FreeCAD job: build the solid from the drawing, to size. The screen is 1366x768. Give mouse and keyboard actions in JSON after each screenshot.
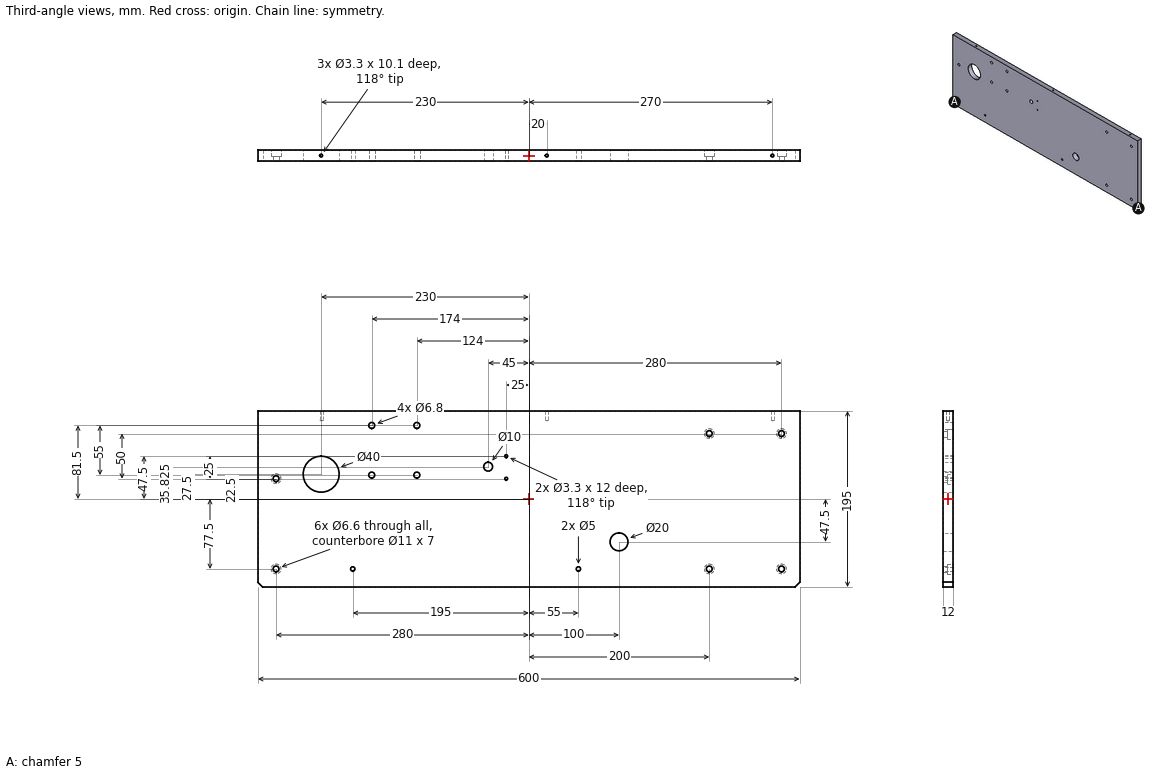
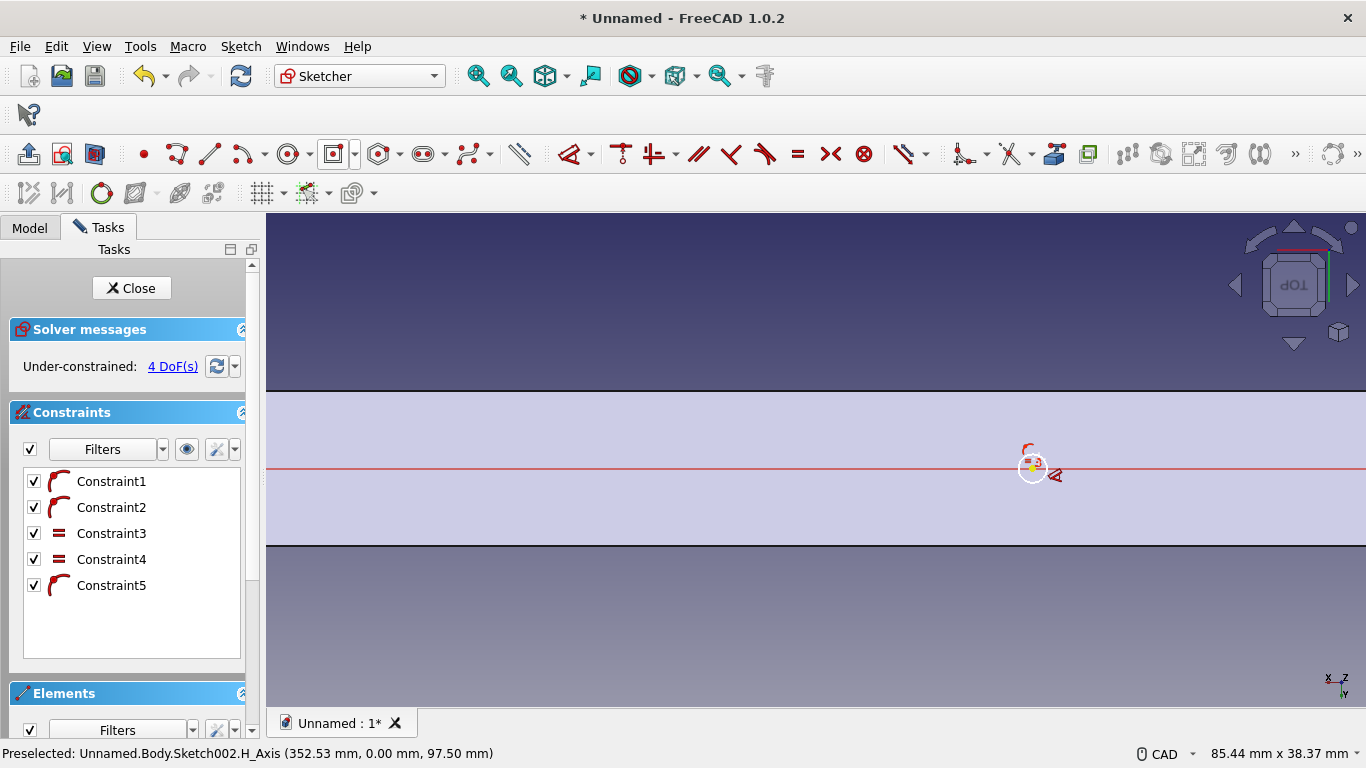
{"action": "left_click", "coordinate": [1033, 454]}
{"action": "left_click", "coordinate": [1034, 422]}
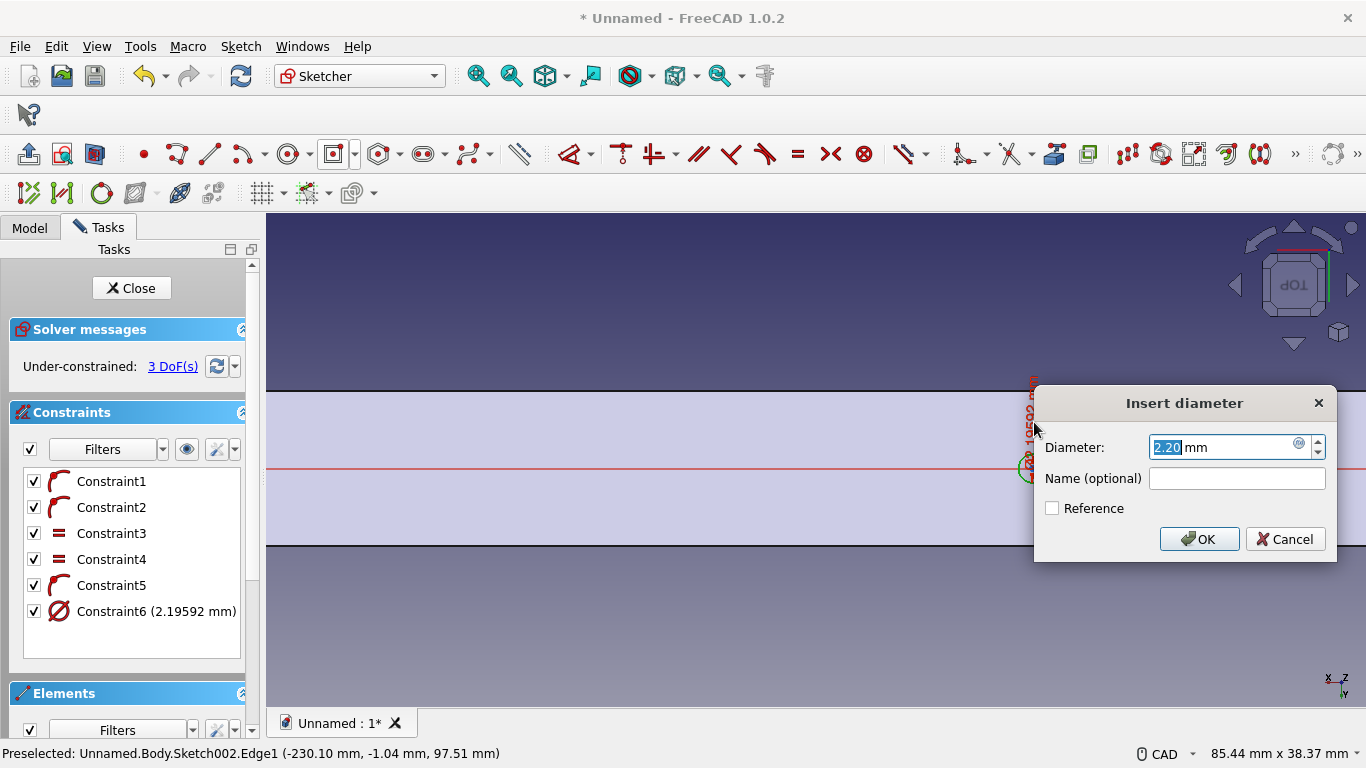
{"action": "type", "text": "3.3"}
{"action": "key", "text": "Return"}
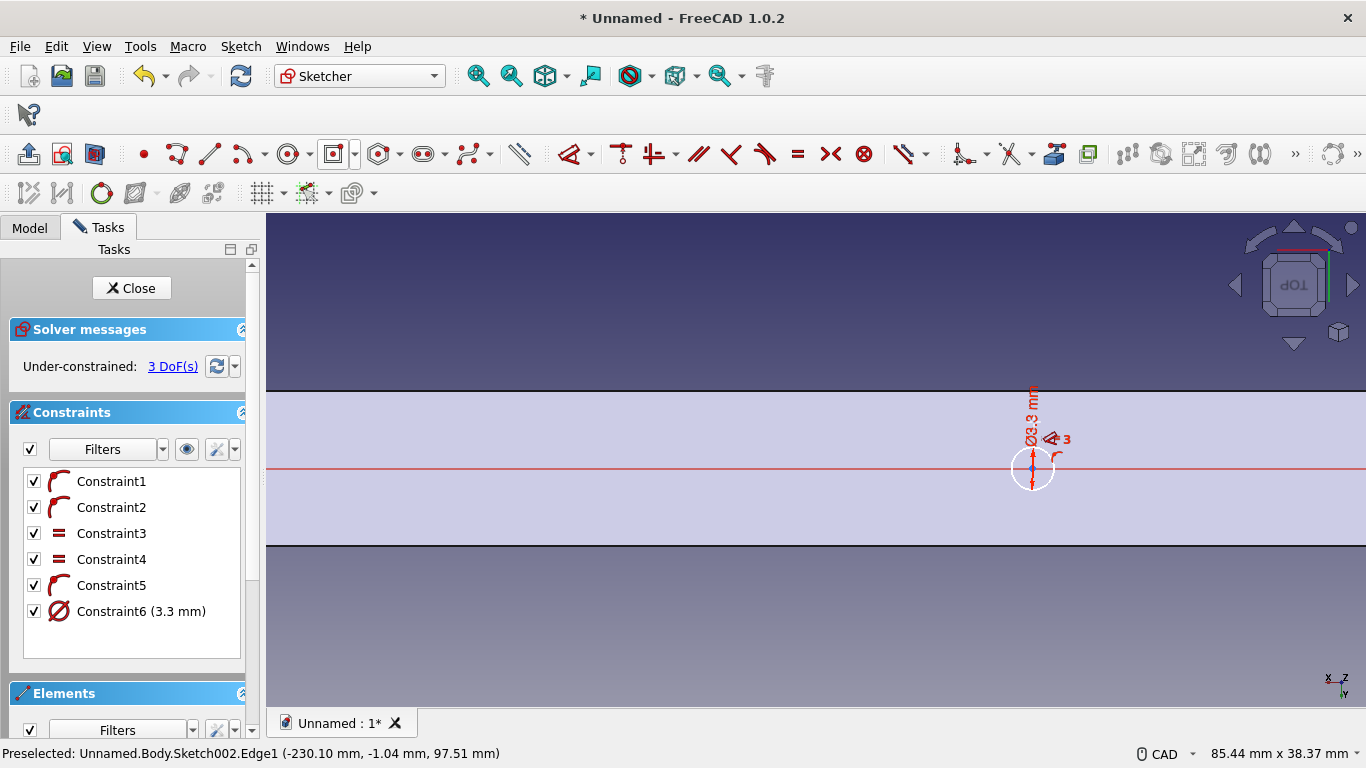
{"action": "scroll", "coordinate": [1040, 459], "scroll_direction": "down", "scroll_amount": 12}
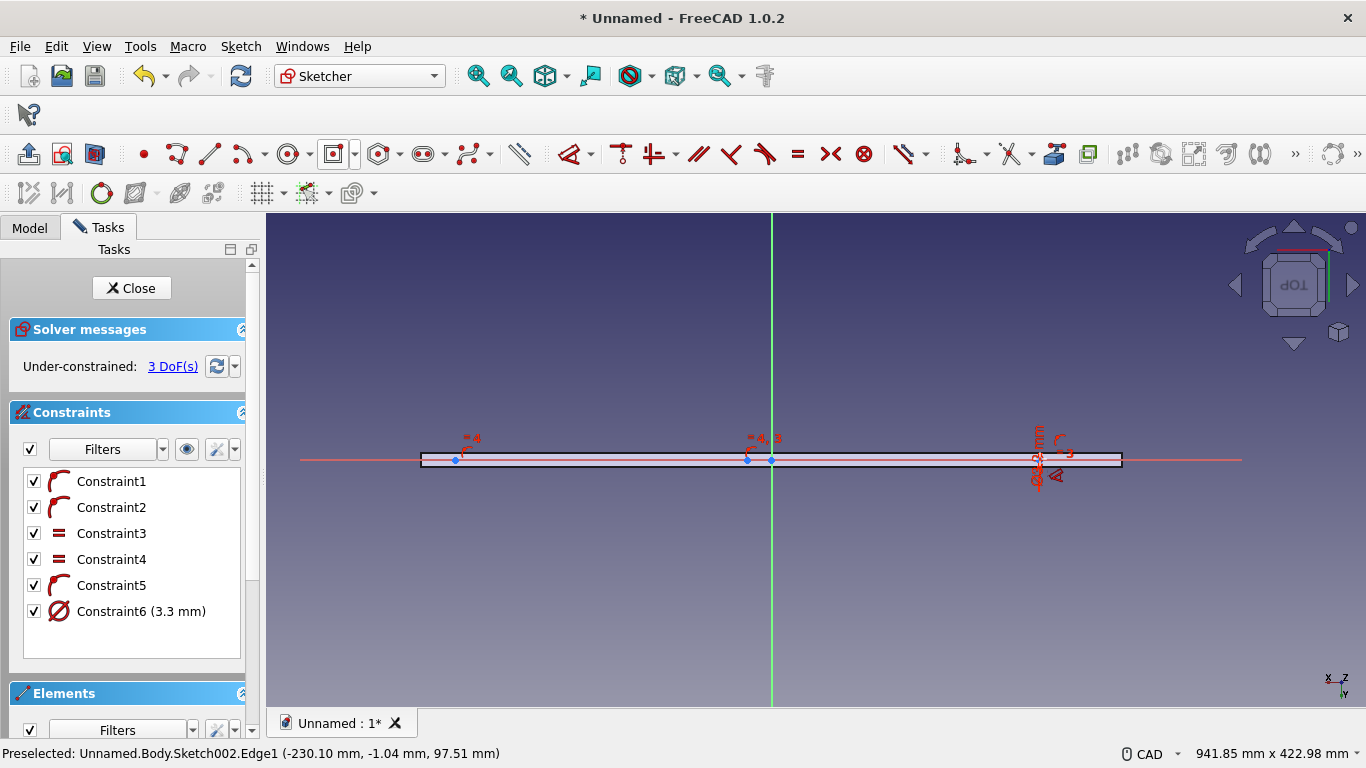
{"action": "scroll", "coordinate": [748, 460], "scroll_direction": "up", "scroll_amount": 3}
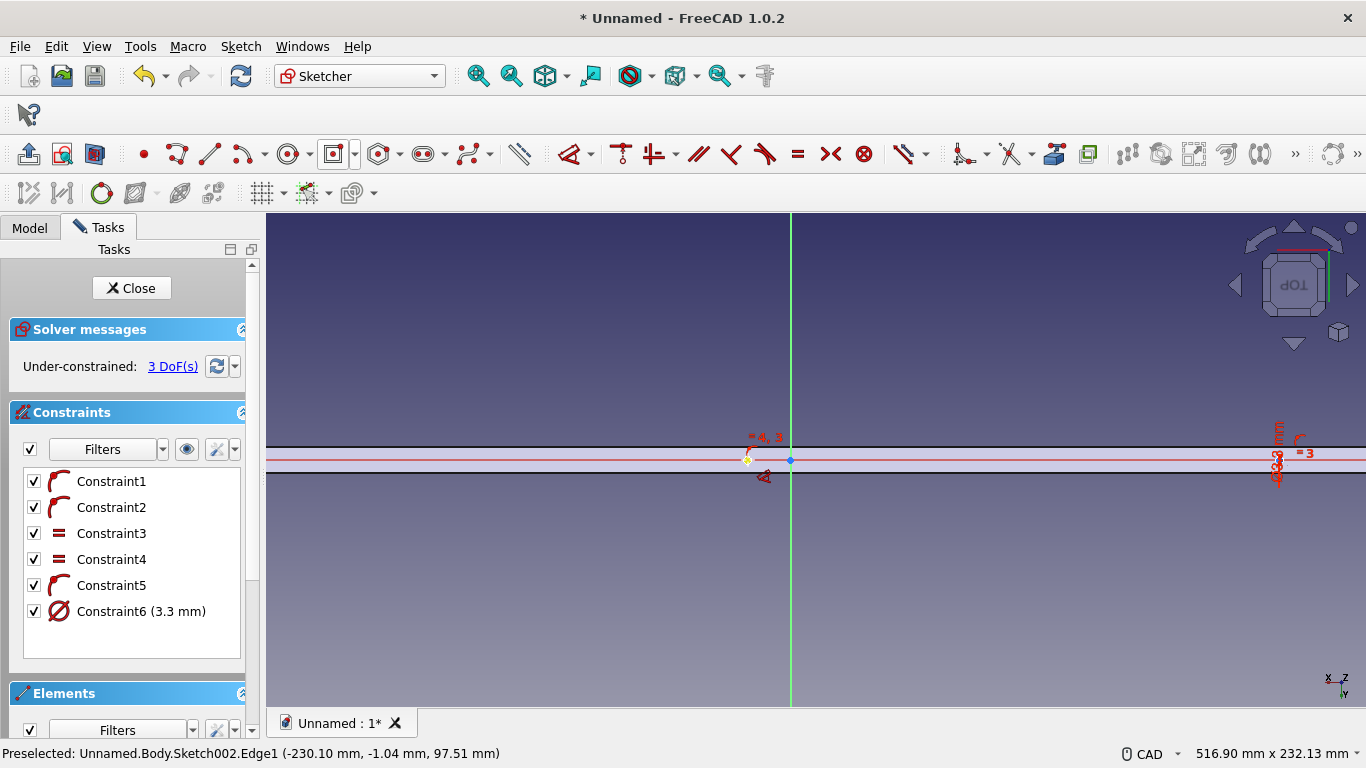
{"action": "left_click", "coordinate": [748, 460]}
{"action": "left_click", "coordinate": [769, 494]}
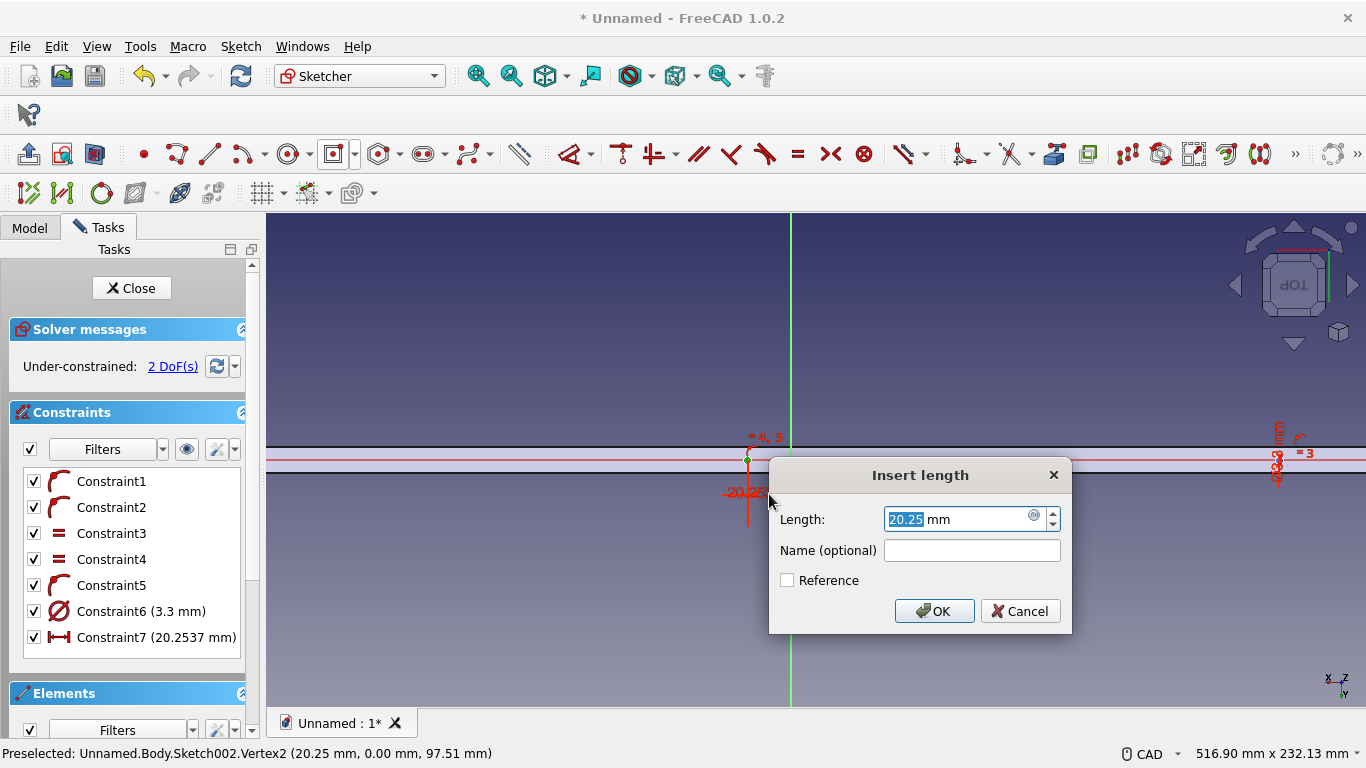
{"action": "type", "text": "20"}
{"action": "key", "text": "Return"}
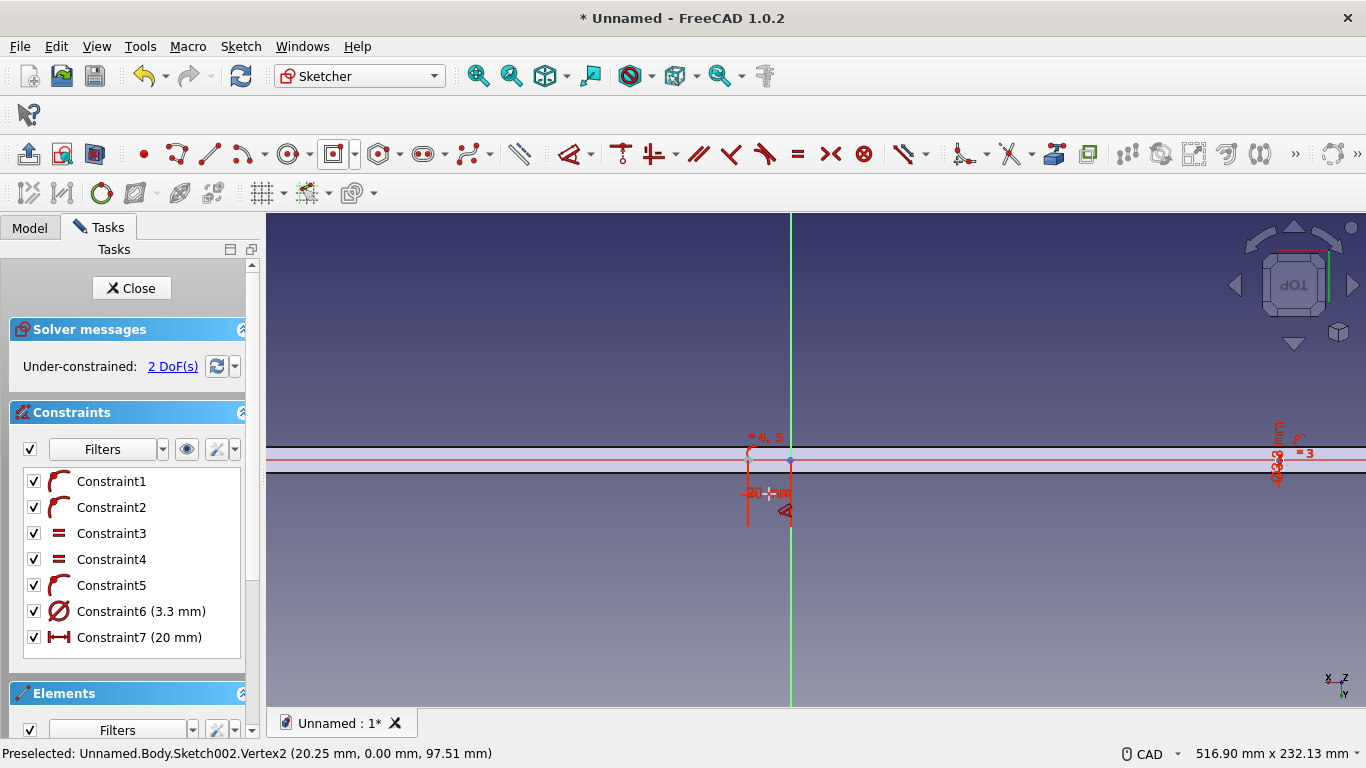
{"action": "scroll", "coordinate": [747, 460], "scroll_direction": "down", "scroll_amount": 3}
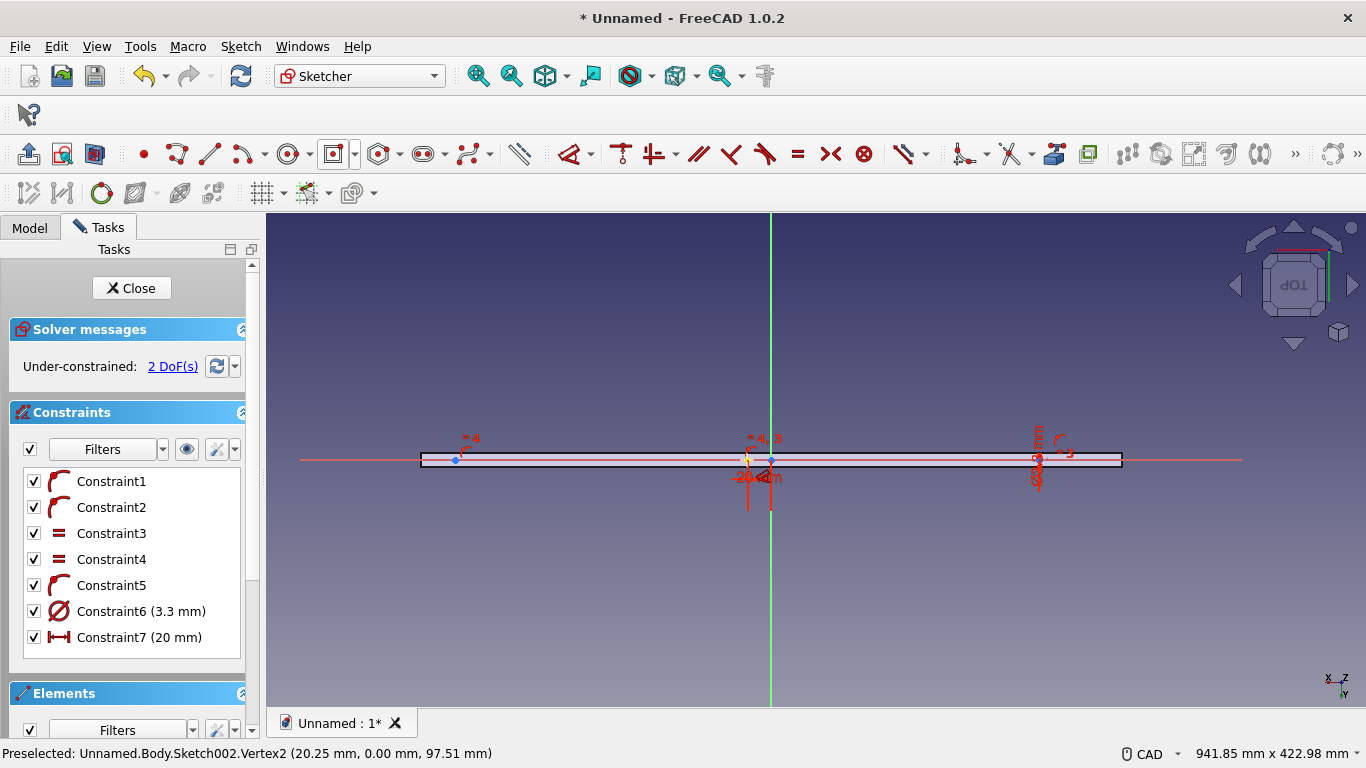
{"action": "left_click", "coordinate": [1040, 460]}
{"action": "left_click", "coordinate": [905, 494]}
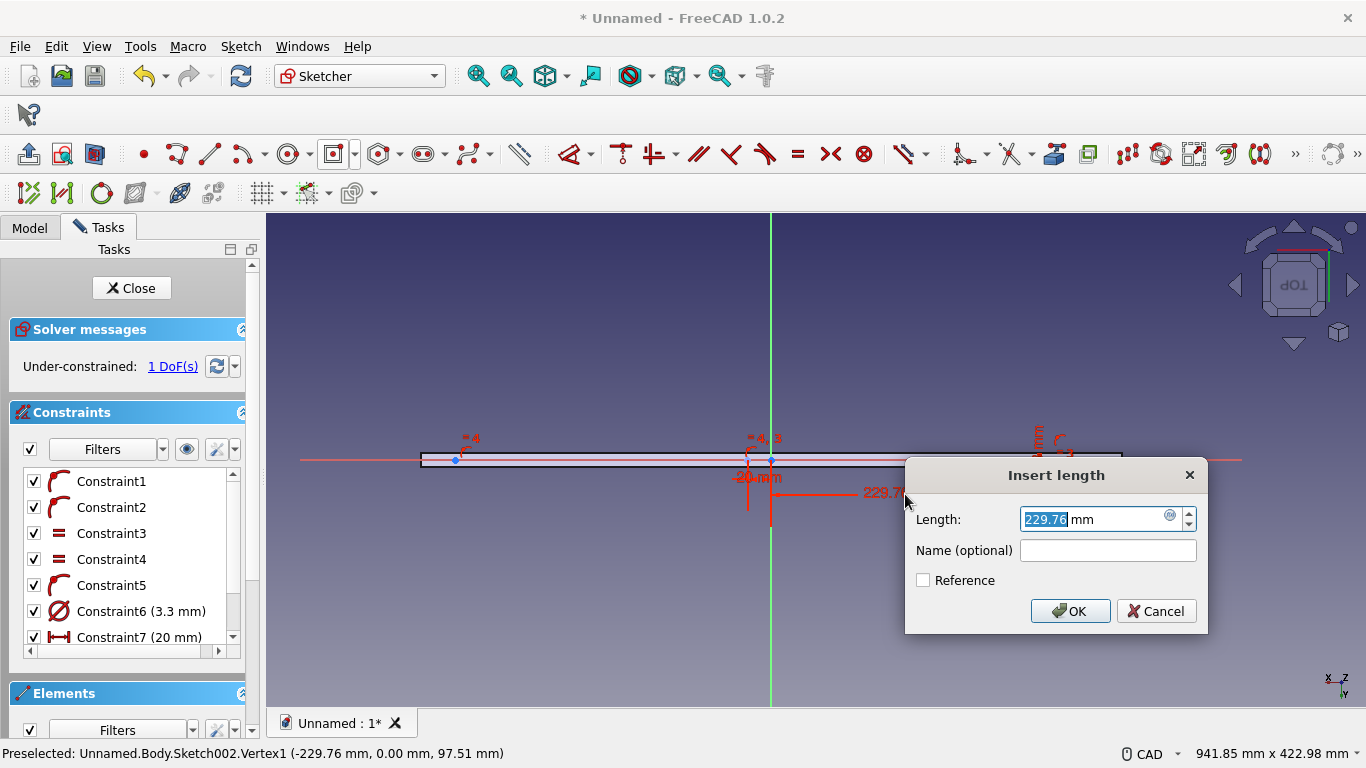
{"action": "type", "text": "230"}
{"action": "key", "text": "Return"}